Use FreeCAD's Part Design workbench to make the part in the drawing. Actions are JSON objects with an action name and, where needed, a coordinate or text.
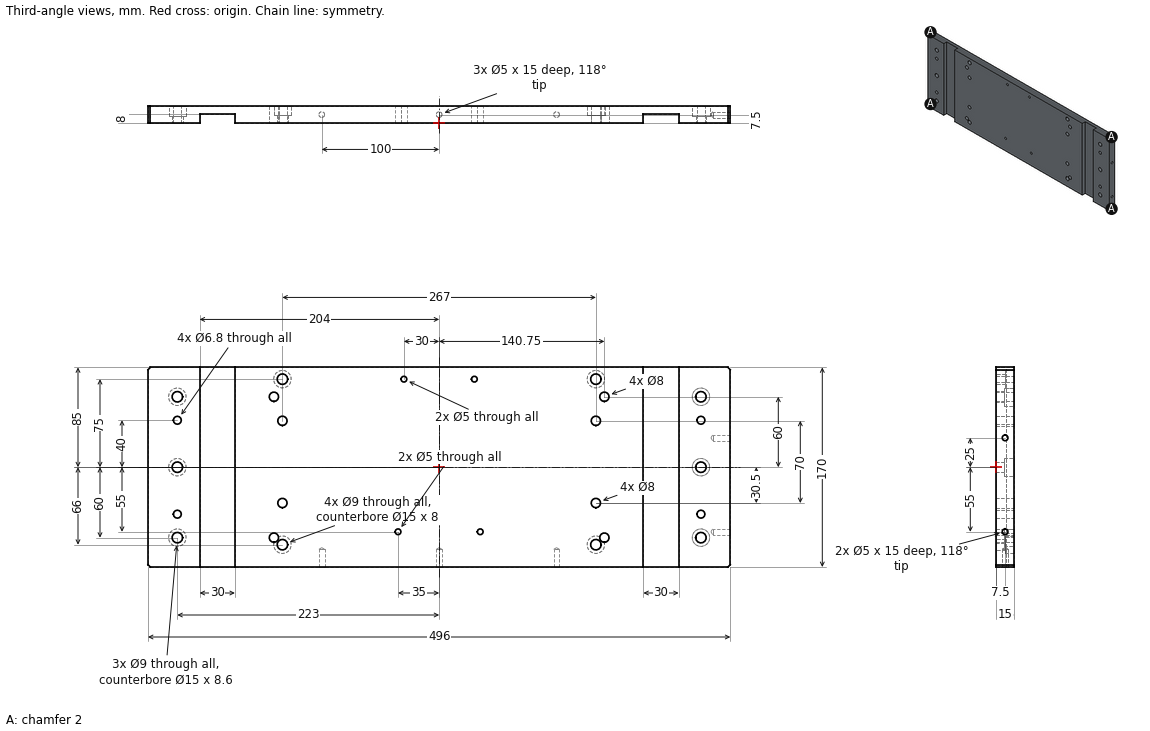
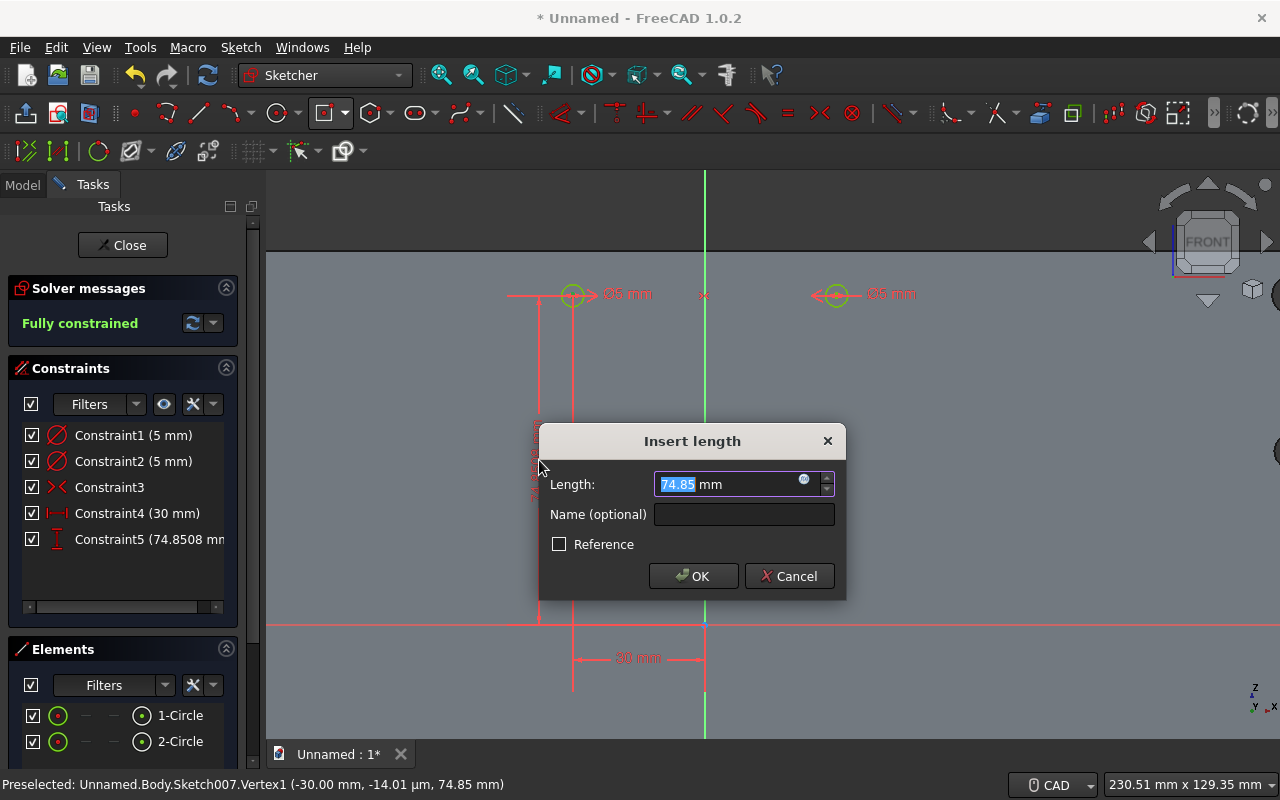
{"action": "type", "text": "75"}
{"action": "key", "text": "Return"}
{"action": "key", "text": "Escape"}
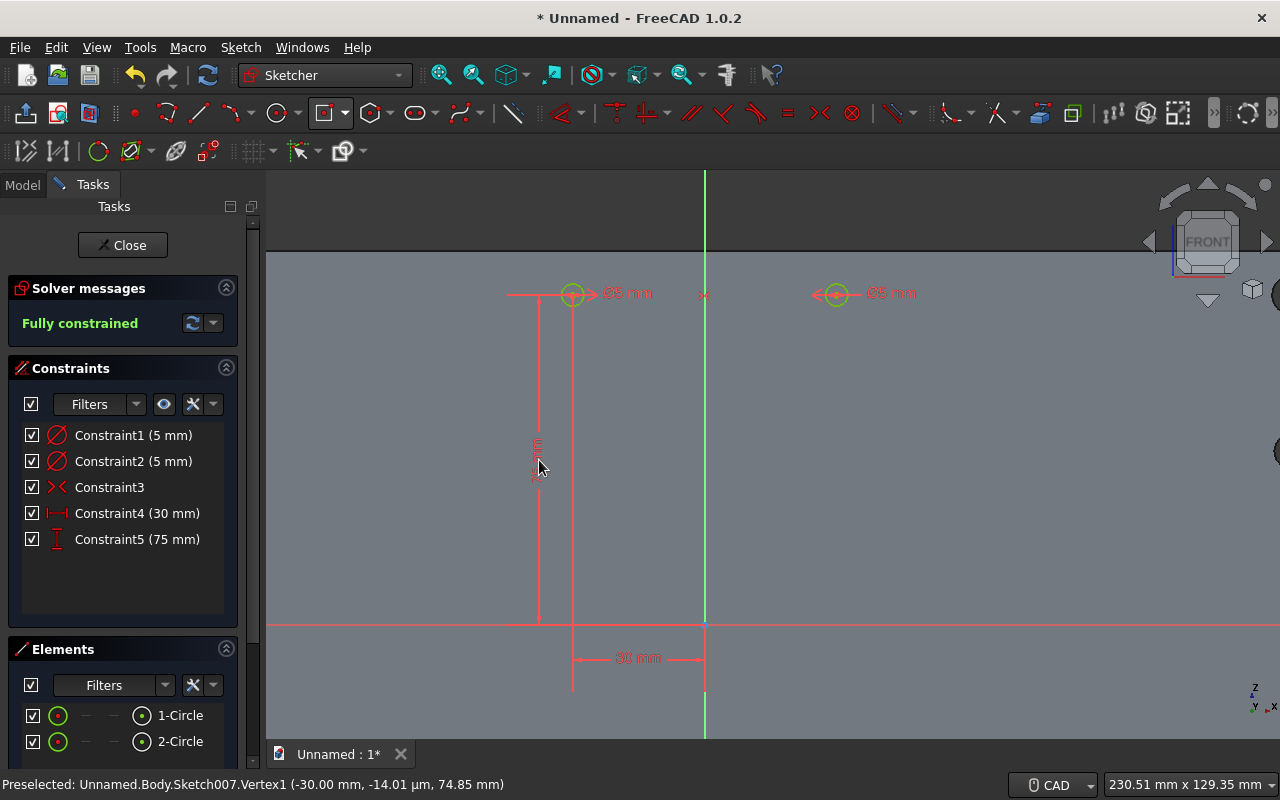
{"action": "left_click", "coordinate": [123, 245]}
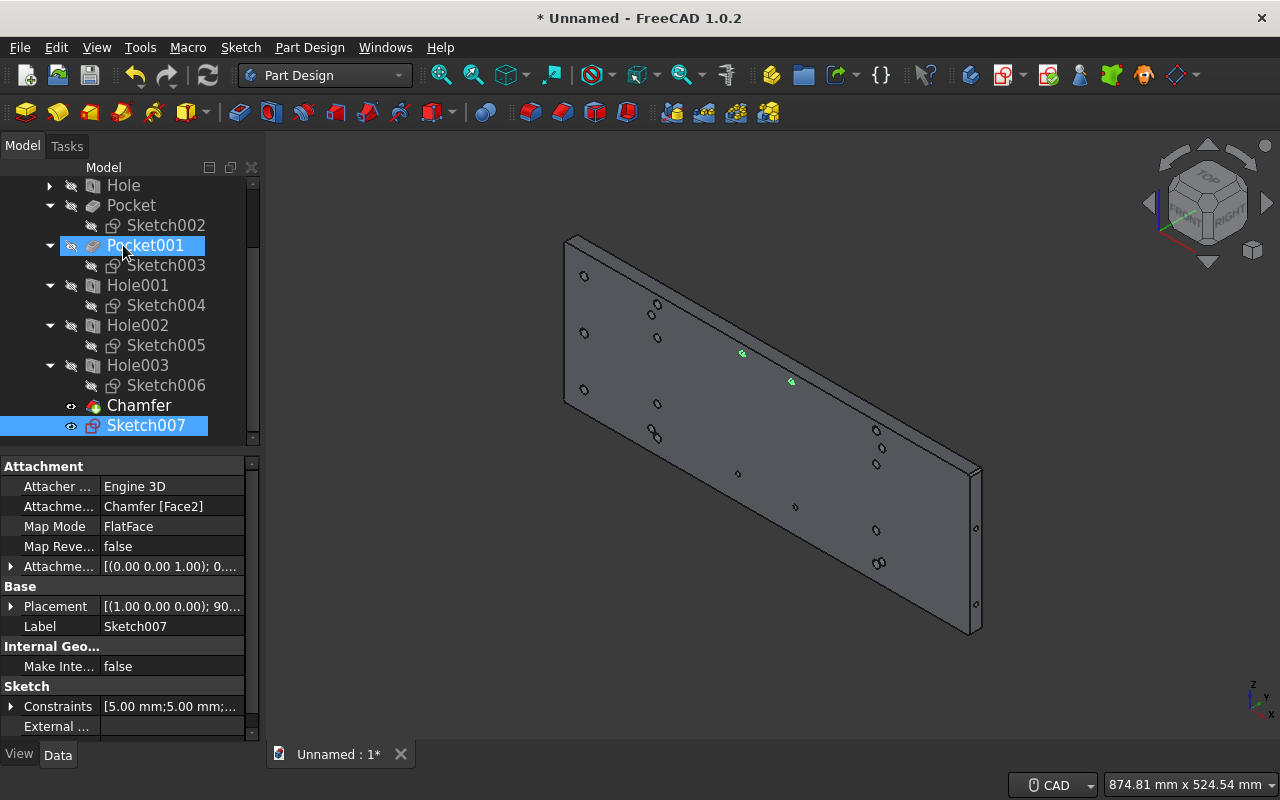
{"action": "left_click", "coordinate": [272, 112]}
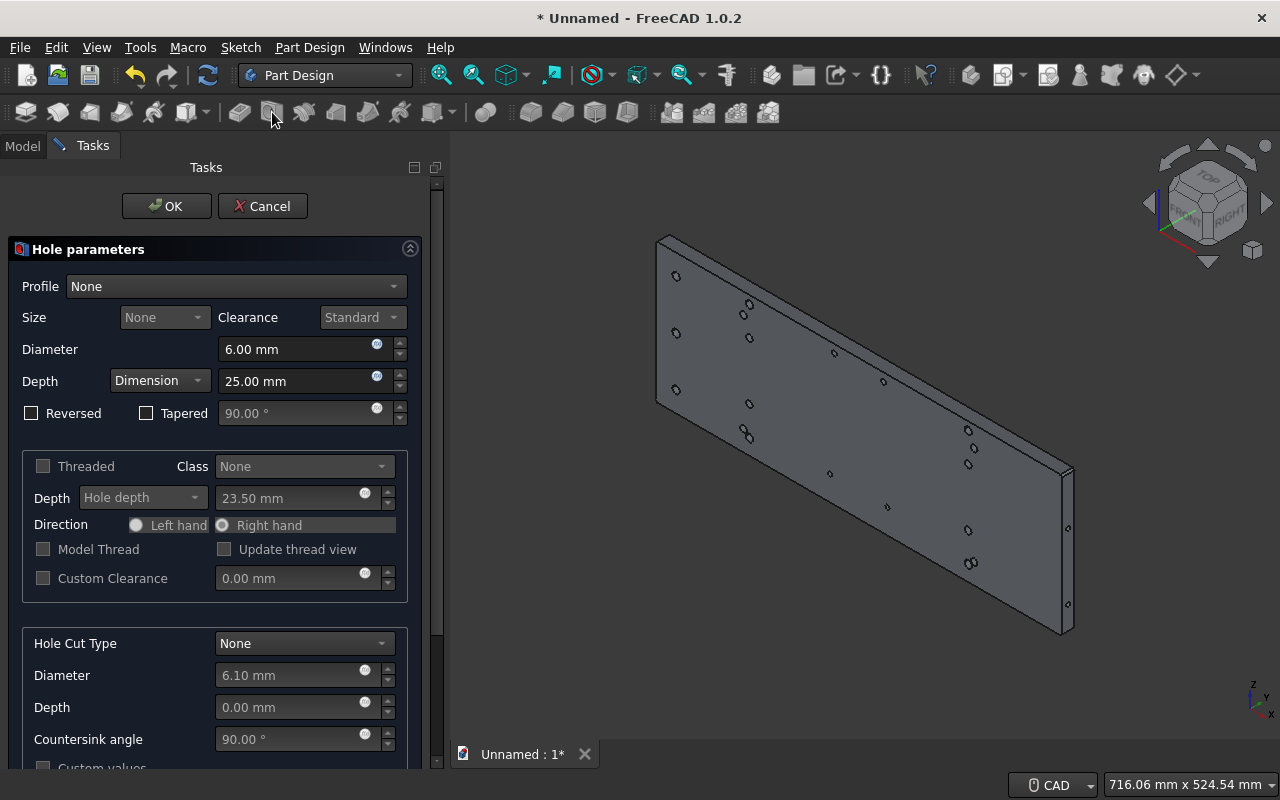
{"action": "triple_click", "coordinate": [305, 349]}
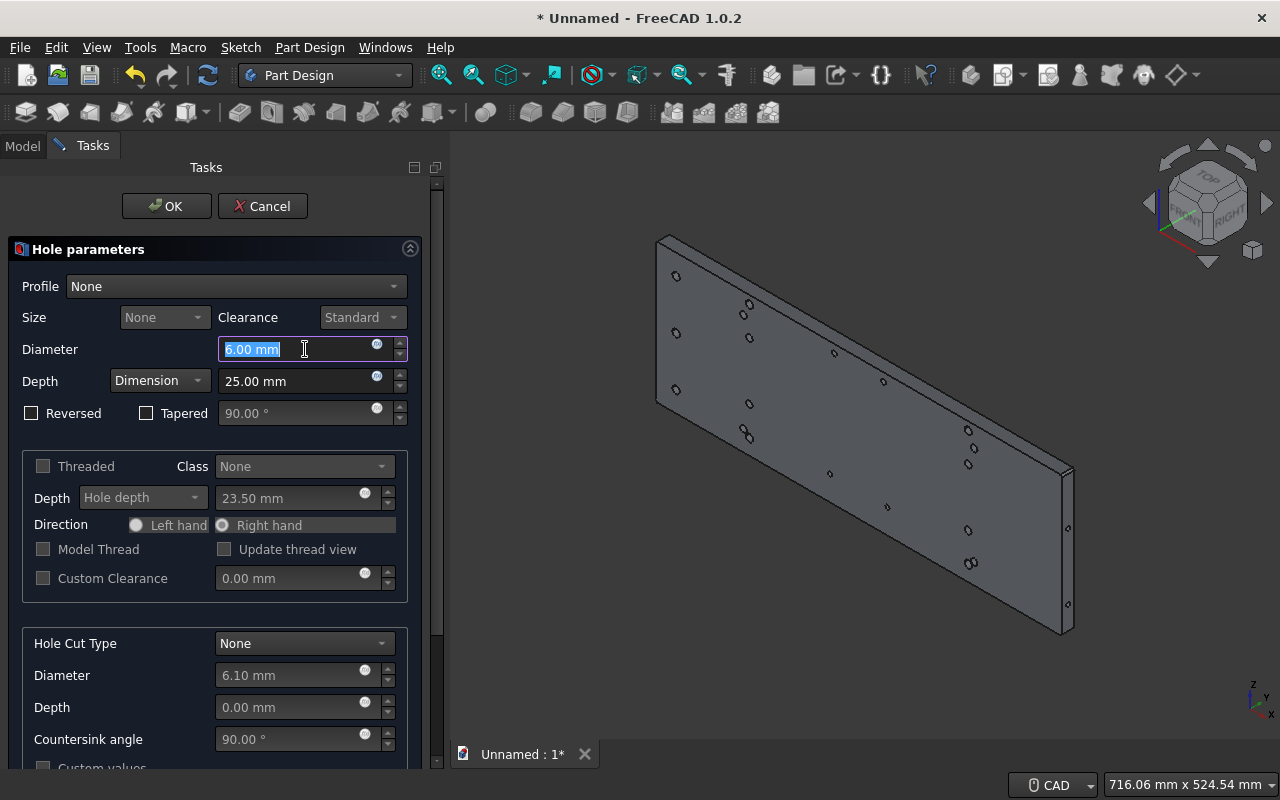
{"action": "type", "text": "5"}
{"action": "key", "text": "Tab"}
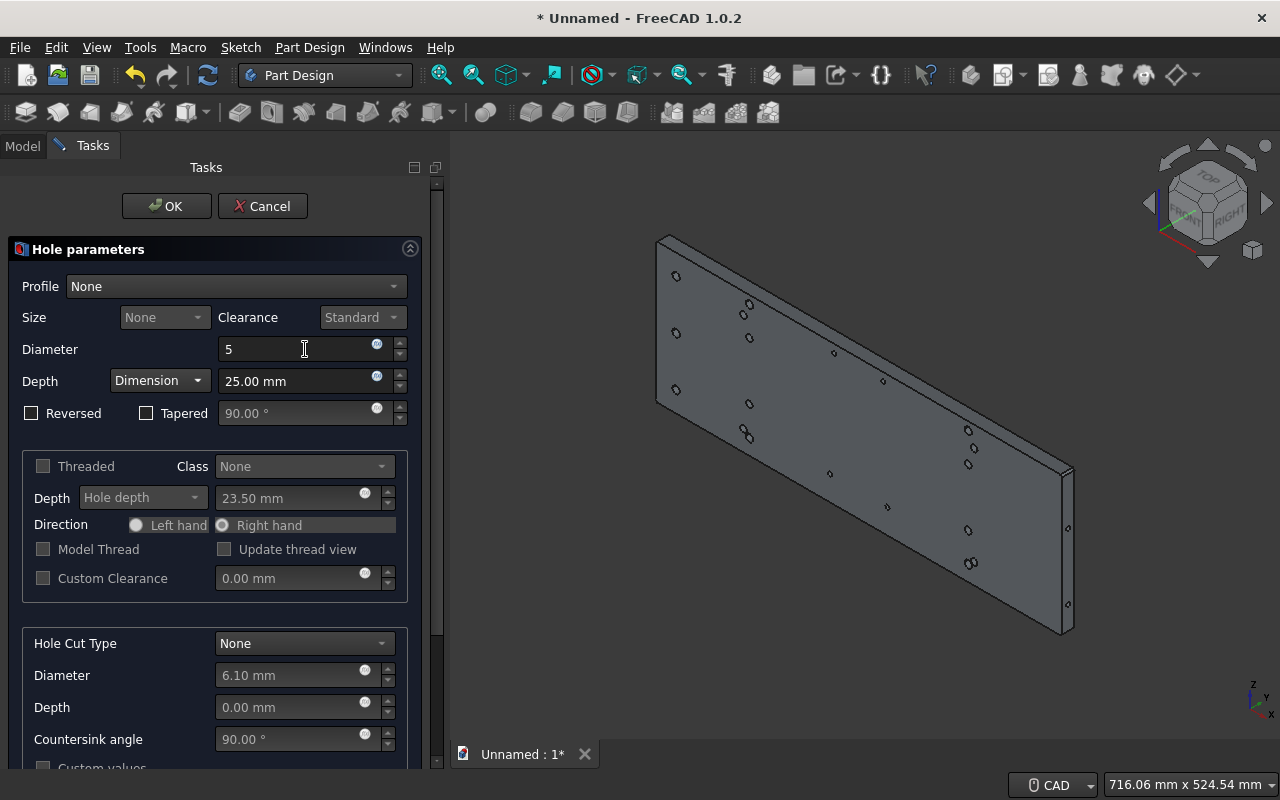
{"action": "left_click", "coordinate": [161, 380]}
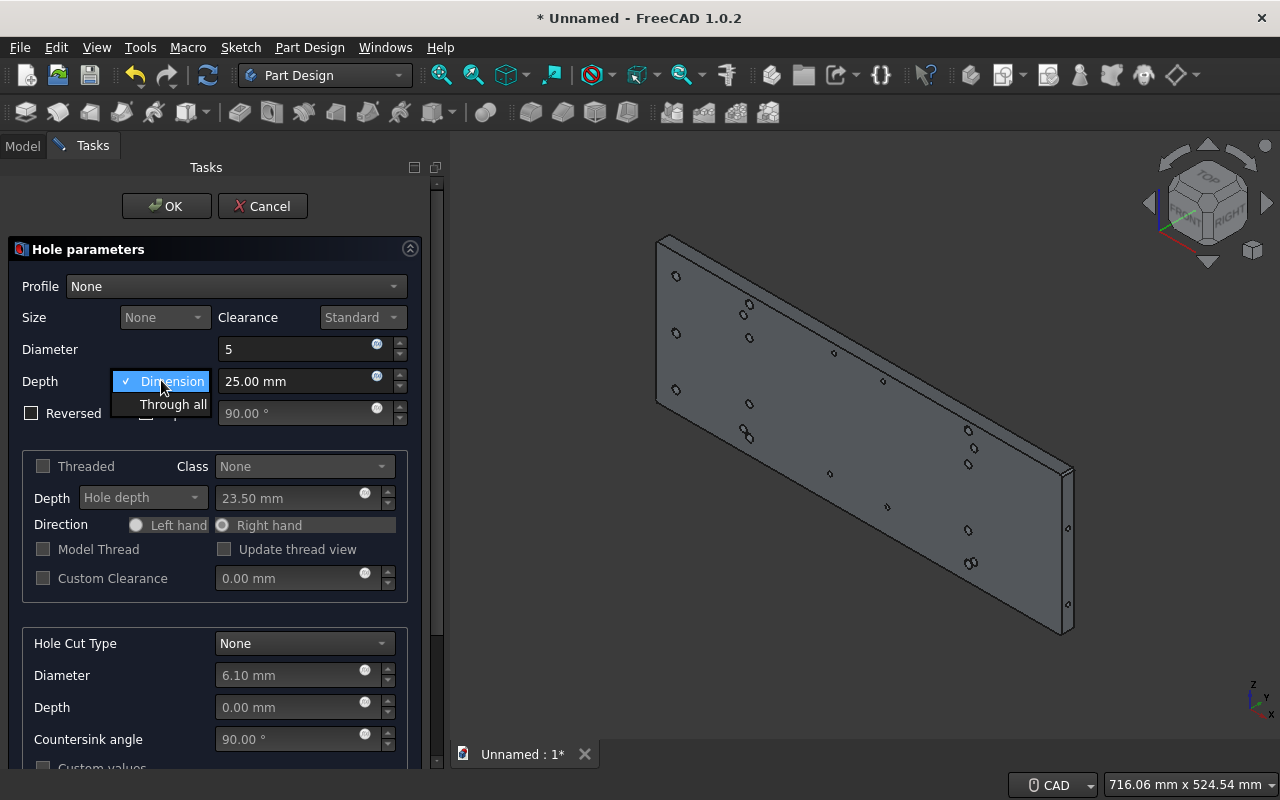
{"action": "left_click", "coordinate": [160, 404]}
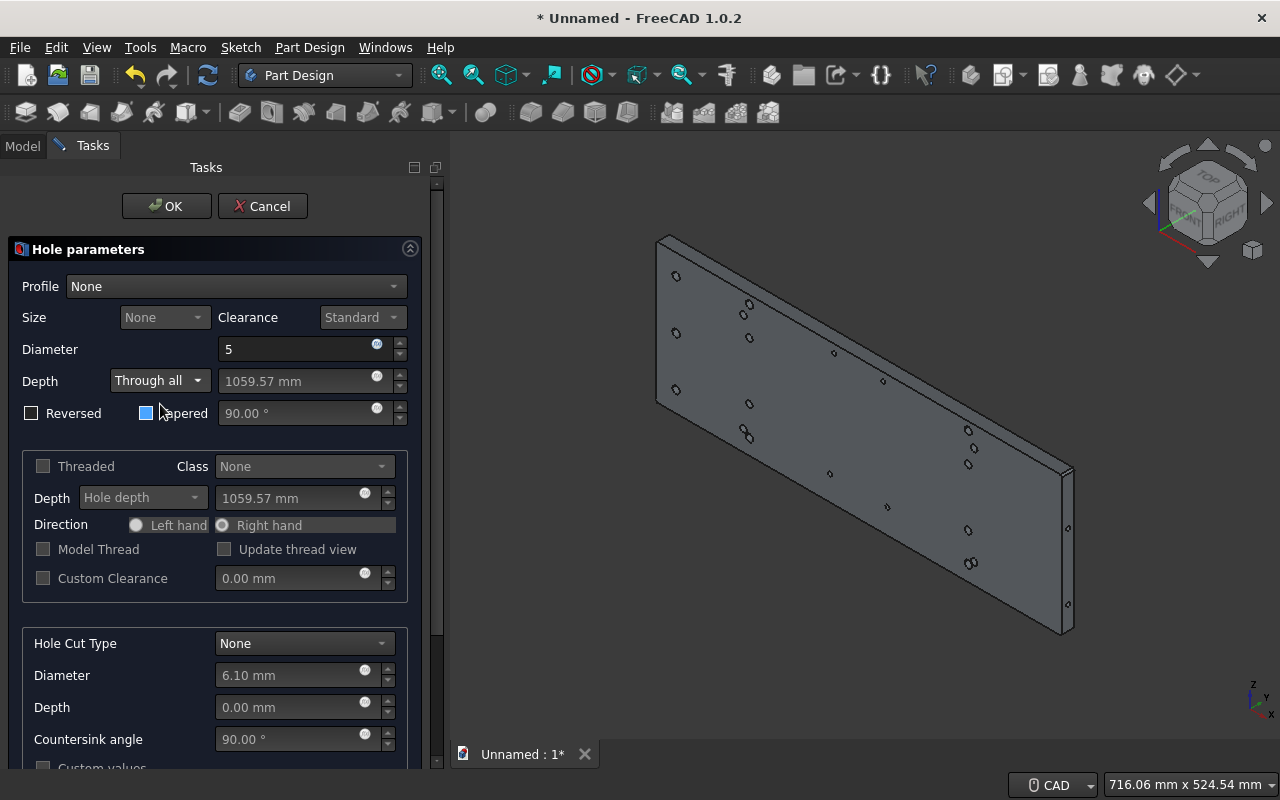
{"action": "left_click", "coordinate": [167, 206]}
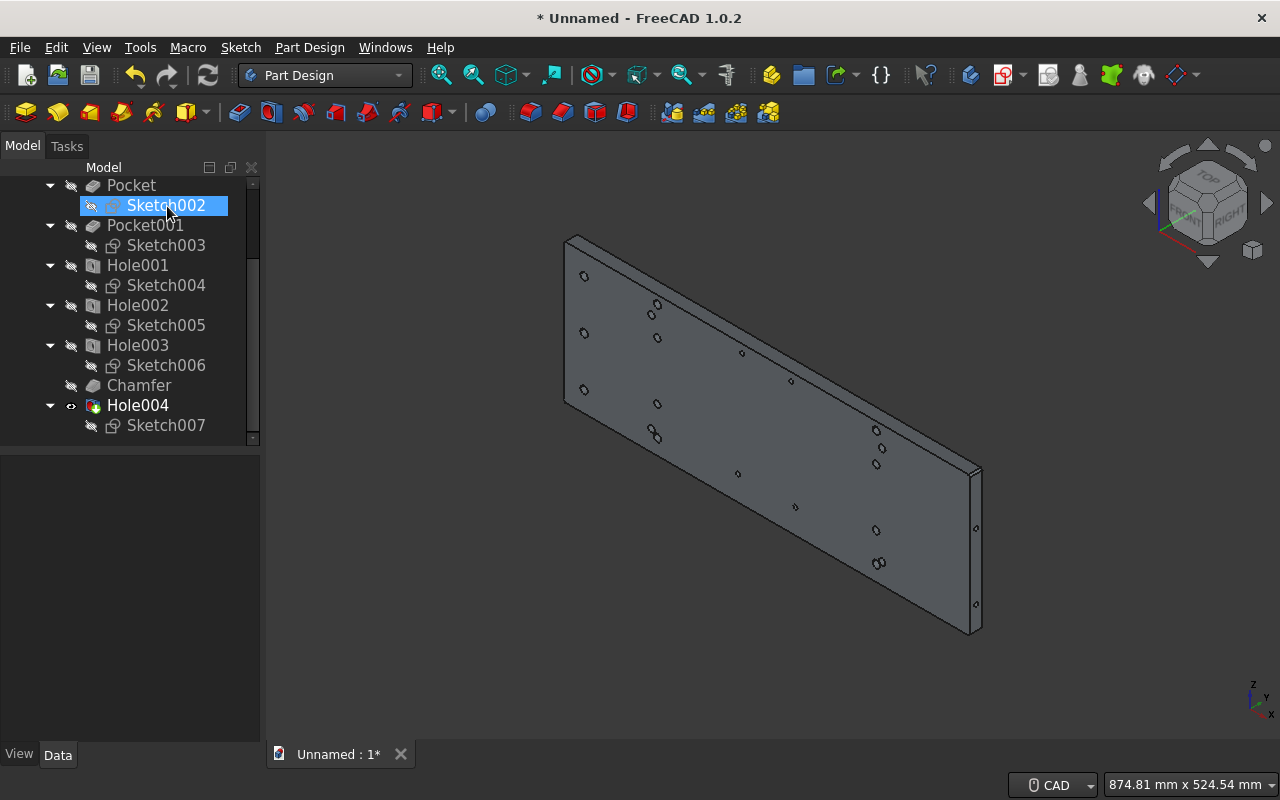
{"action": "key", "text": "5"}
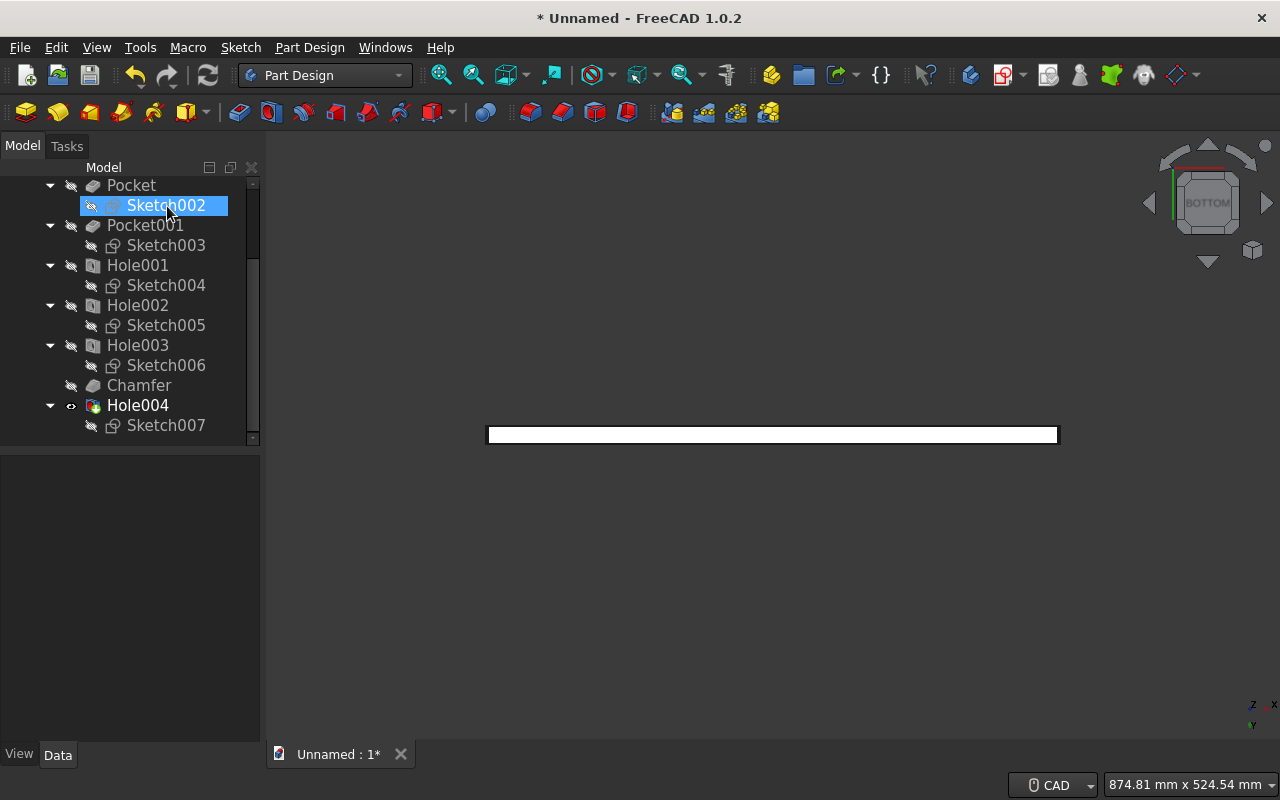
{"action": "left_click", "coordinate": [1017, 434]}